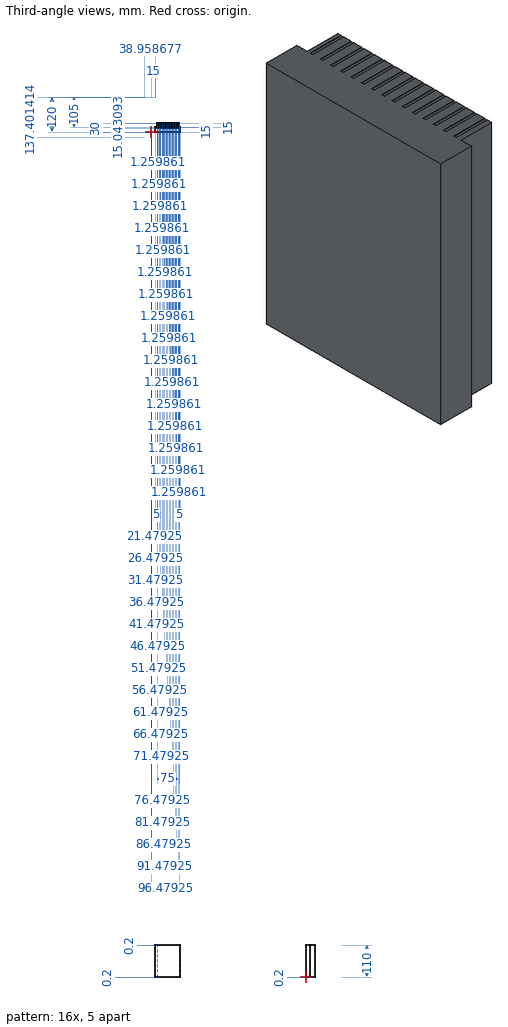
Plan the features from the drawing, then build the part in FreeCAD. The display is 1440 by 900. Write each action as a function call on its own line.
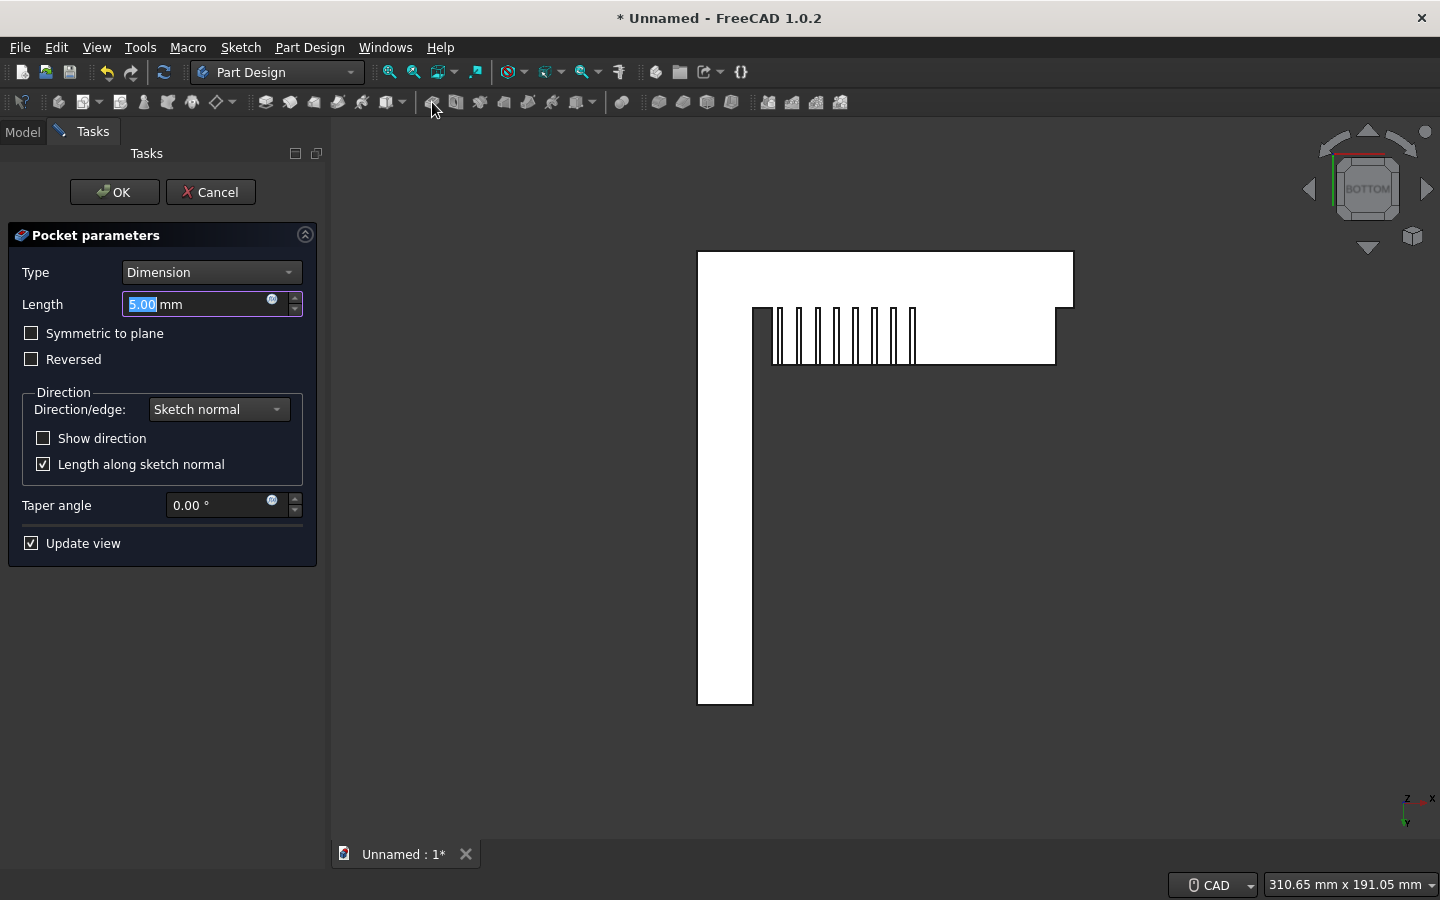
text(0.2)
key(Tab)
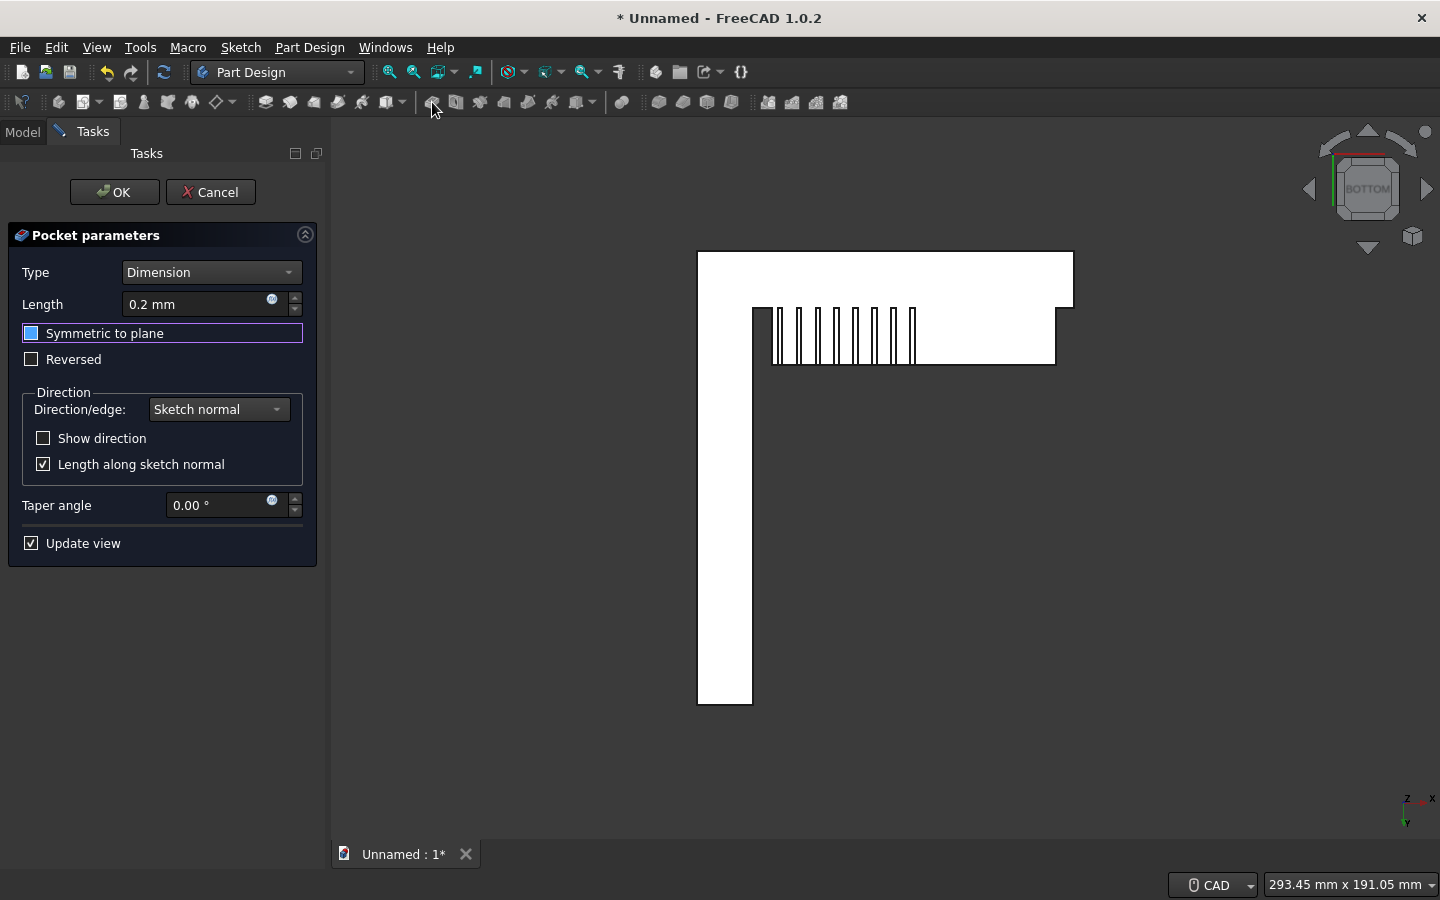
click(115, 192)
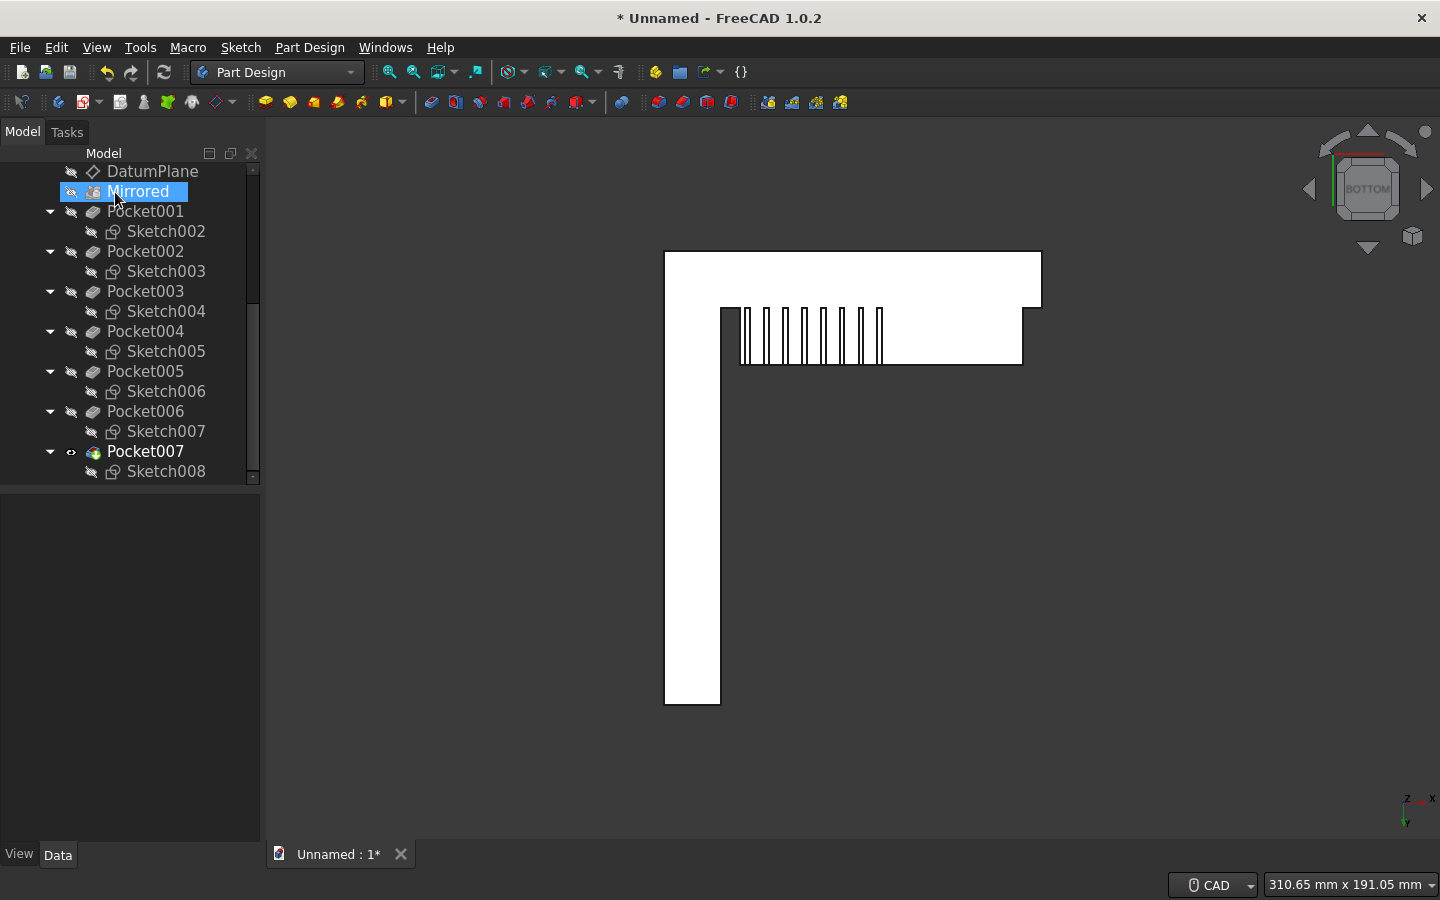
click(84, 102)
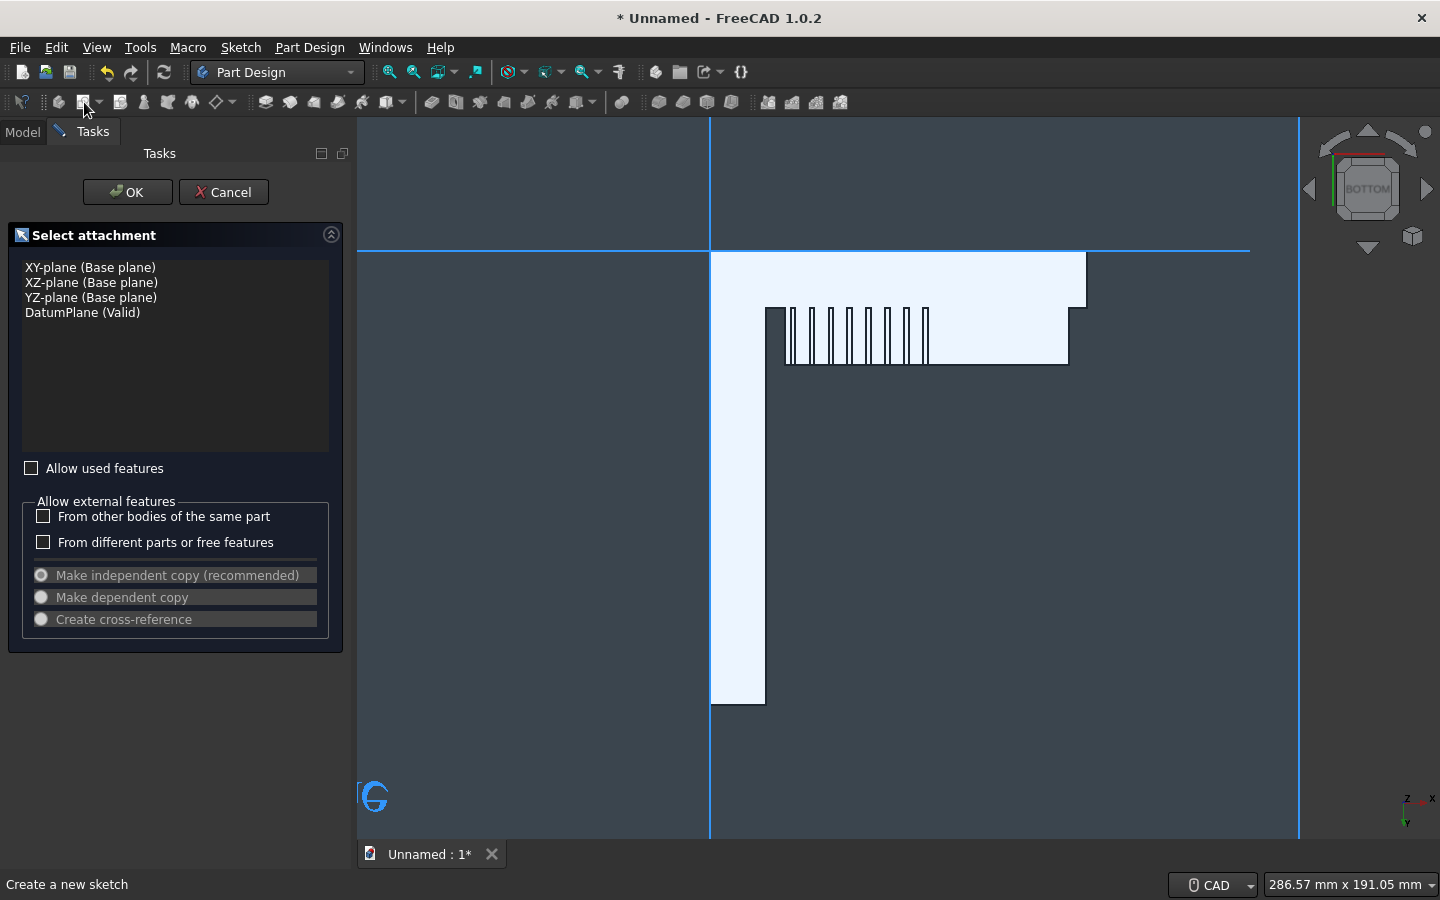
click(82, 268)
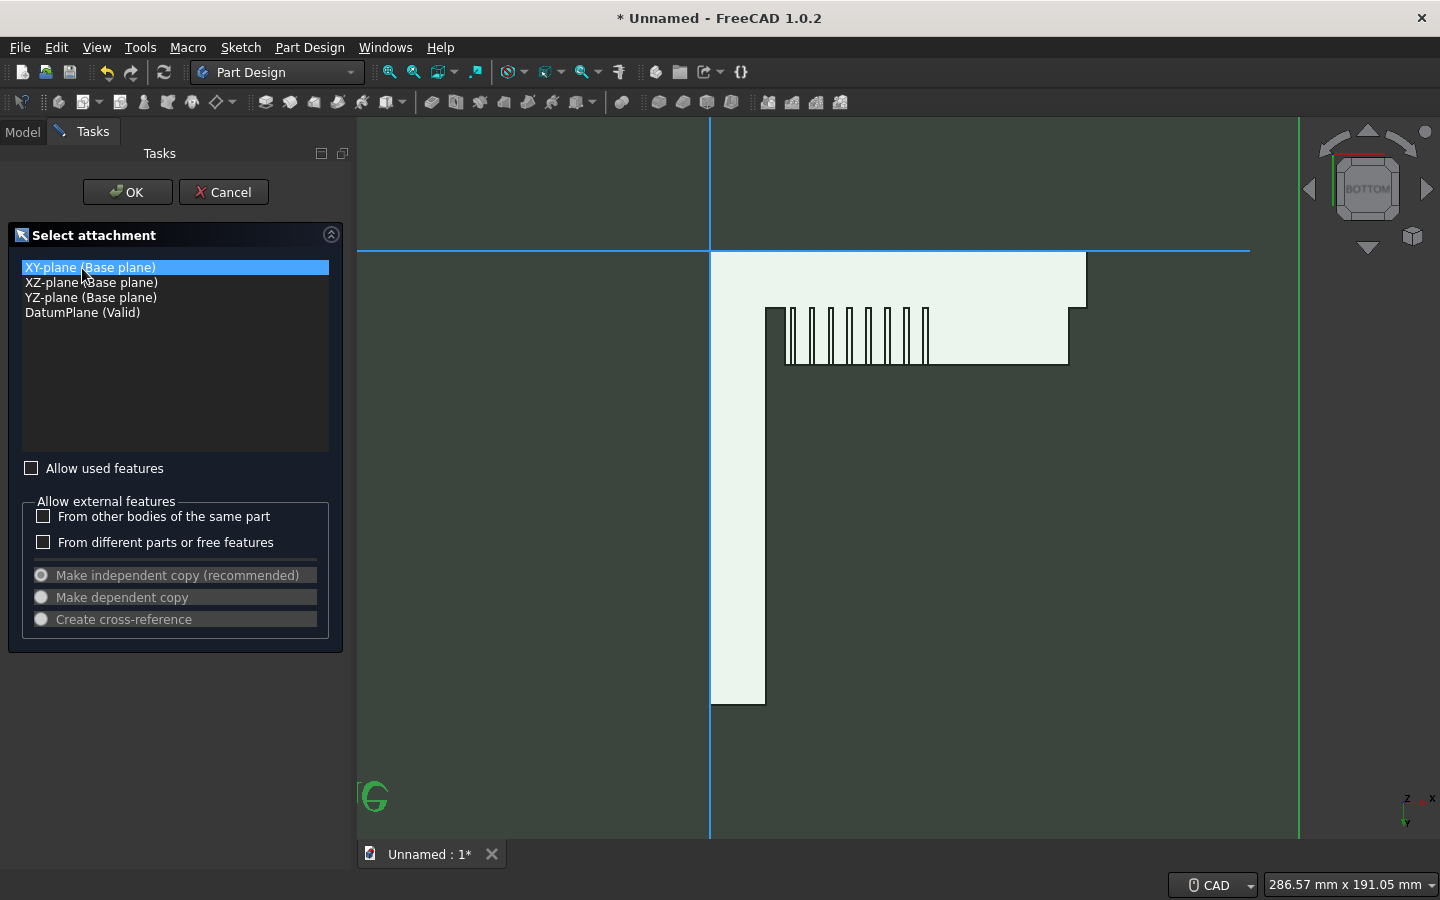
click(128, 192)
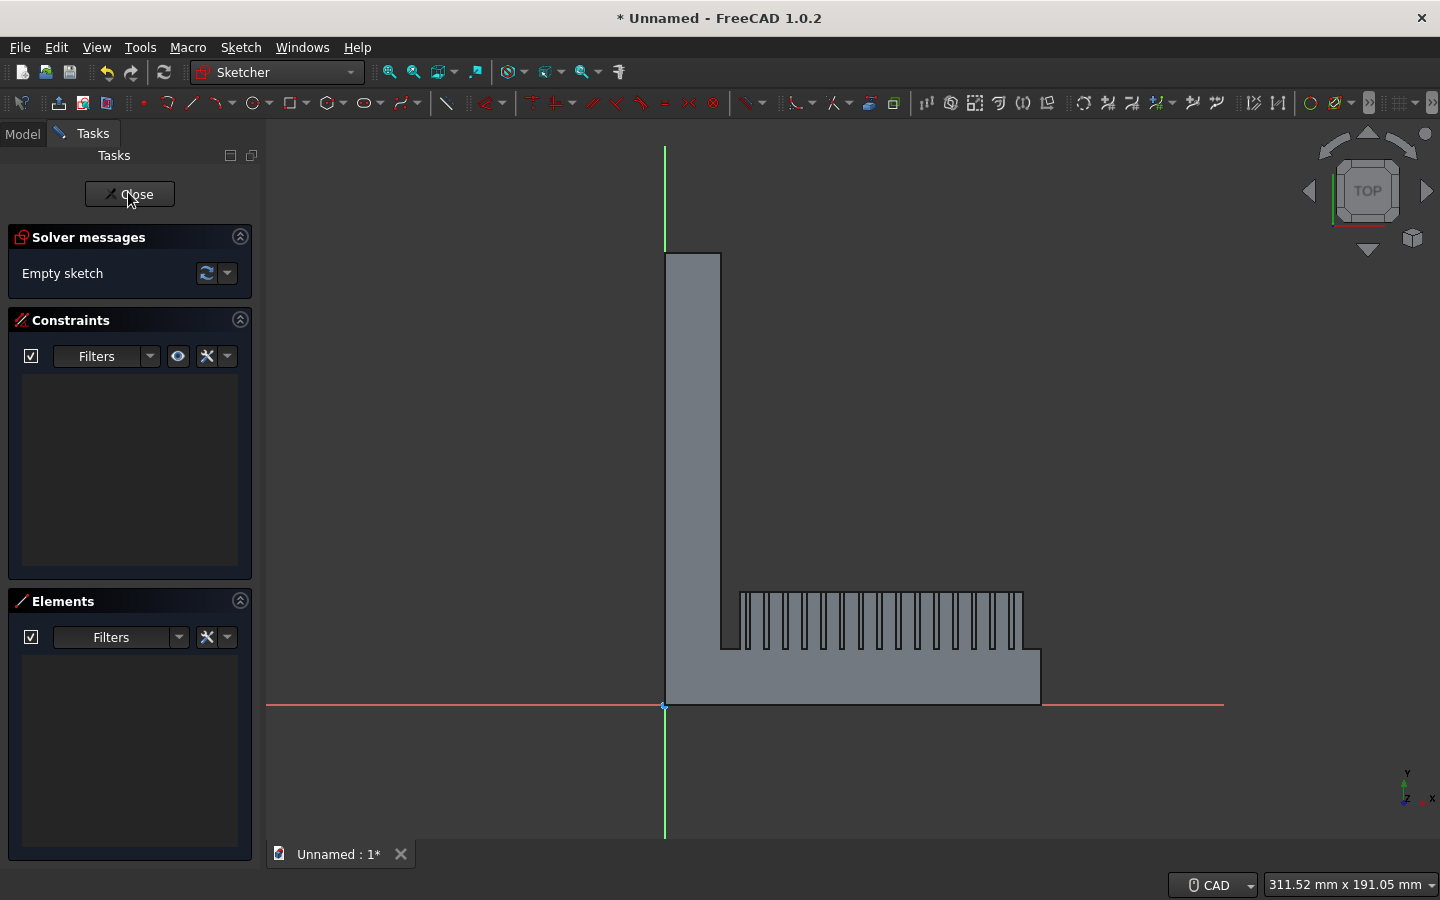
click(108, 104)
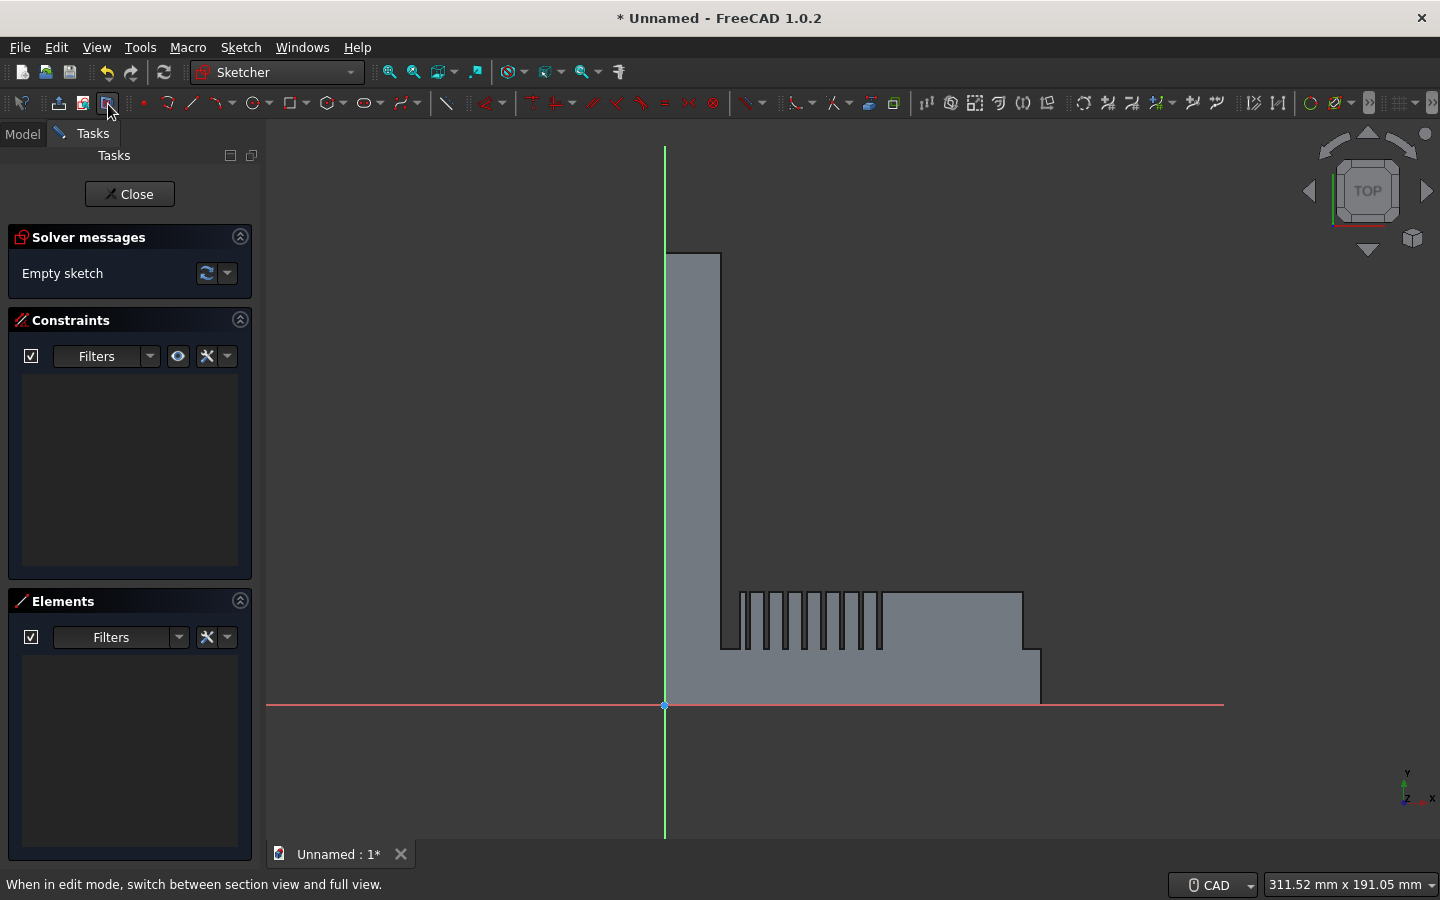
scroll(913, 638, up, 11)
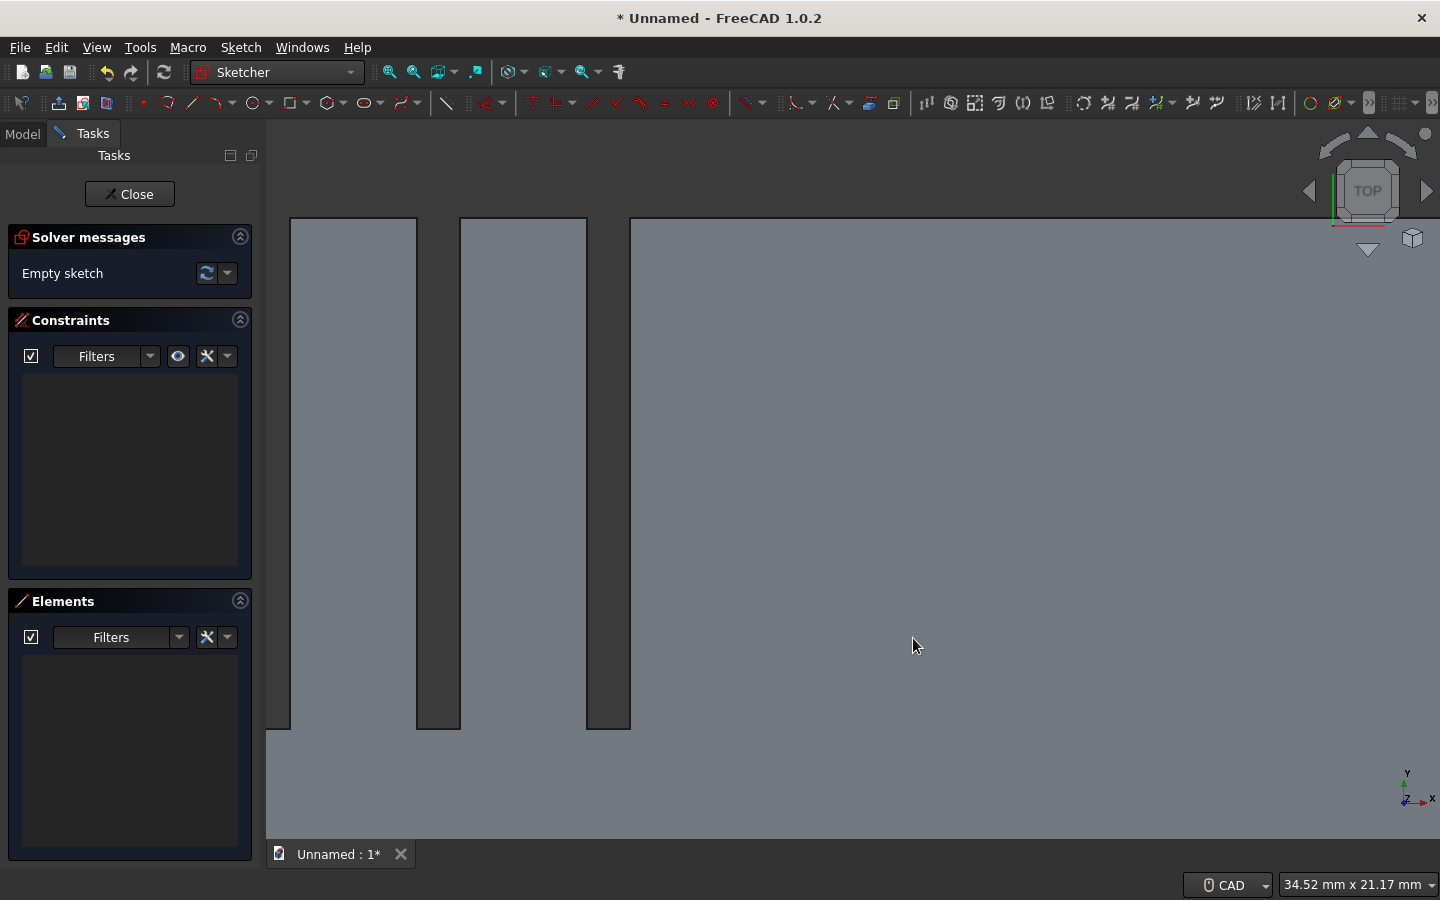
click(290, 104)